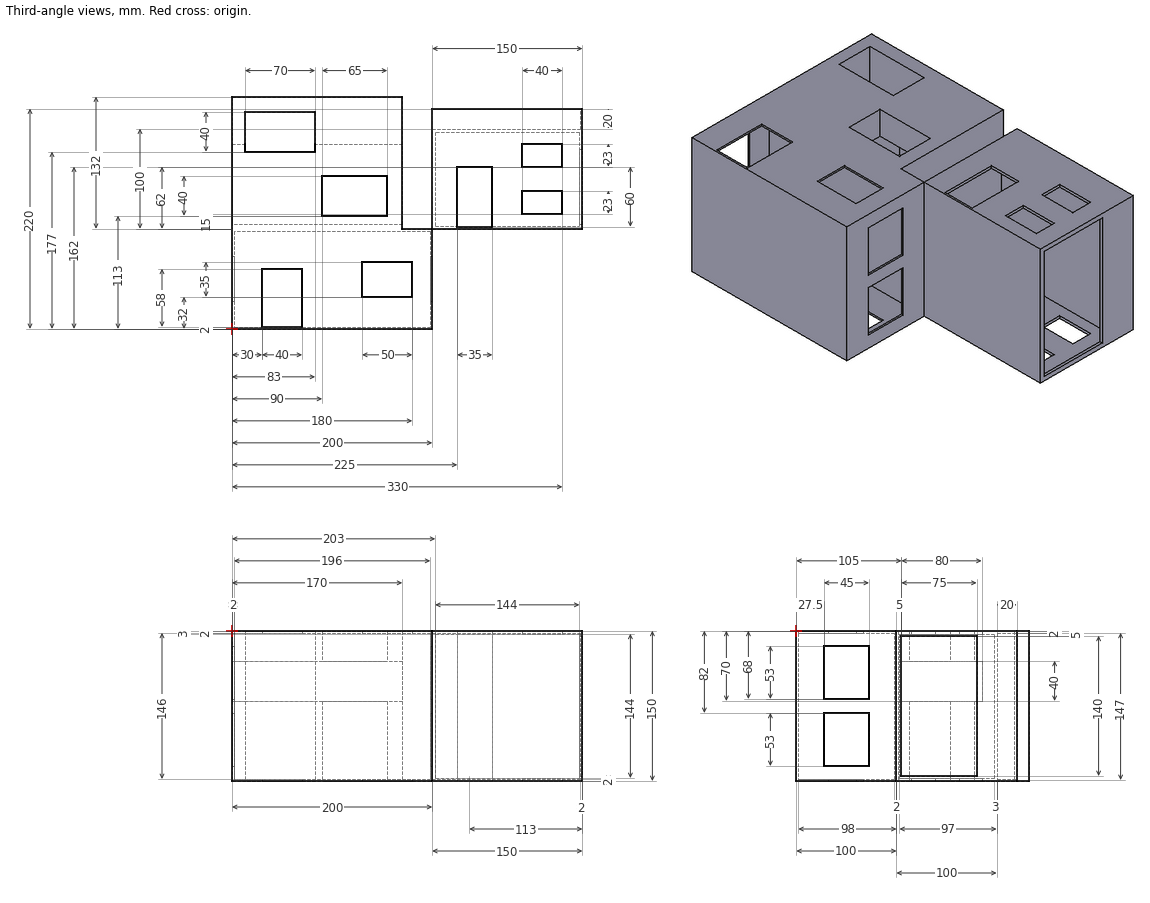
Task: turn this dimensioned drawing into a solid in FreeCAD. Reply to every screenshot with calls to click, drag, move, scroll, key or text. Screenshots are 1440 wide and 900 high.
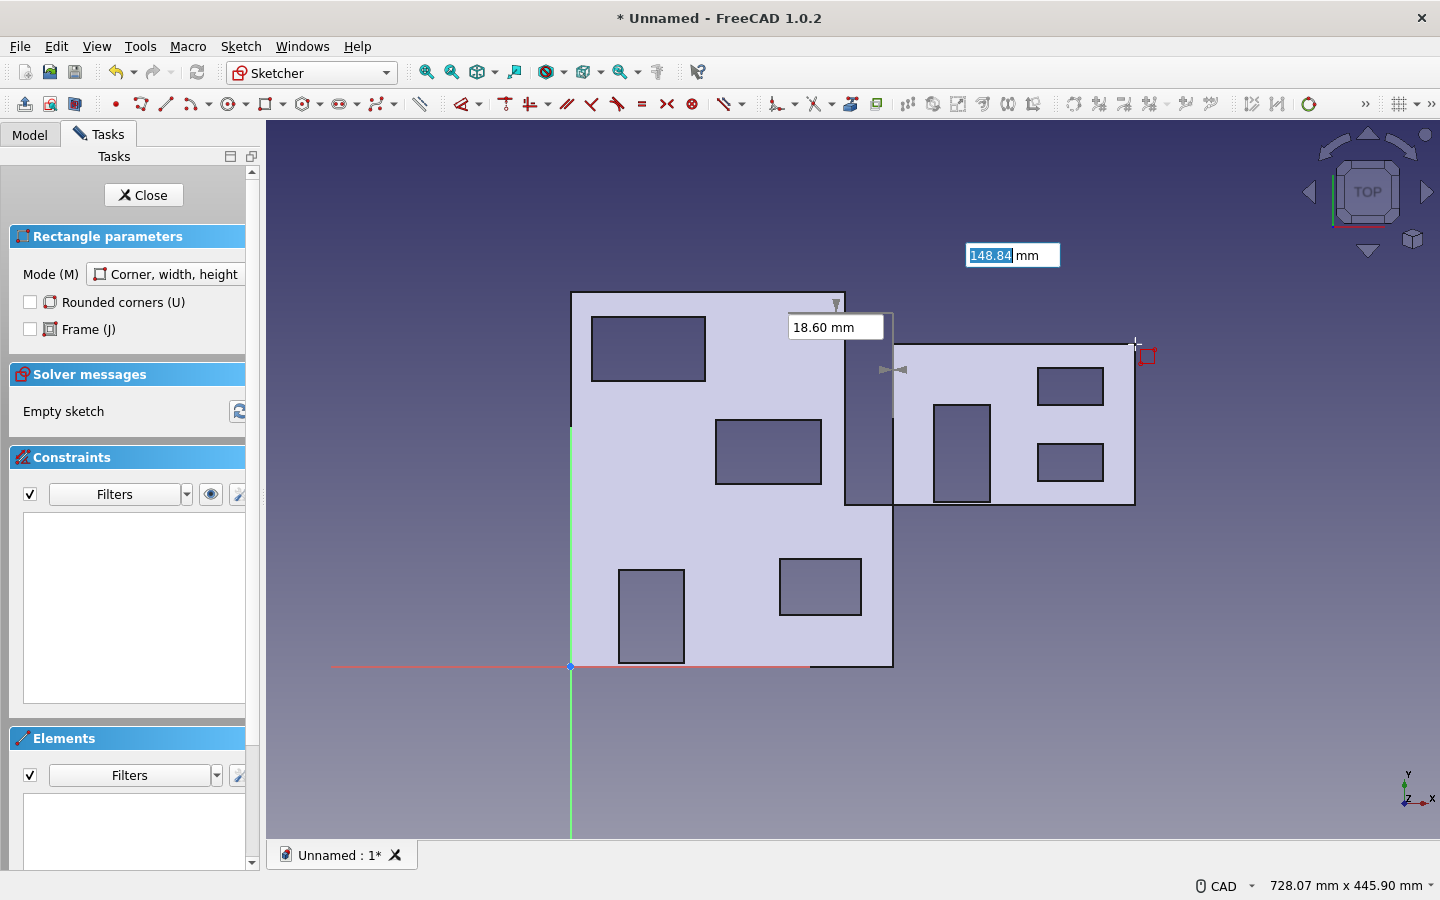
text(150)
key(Tab)
text(20)
key(Return)
key(Escape)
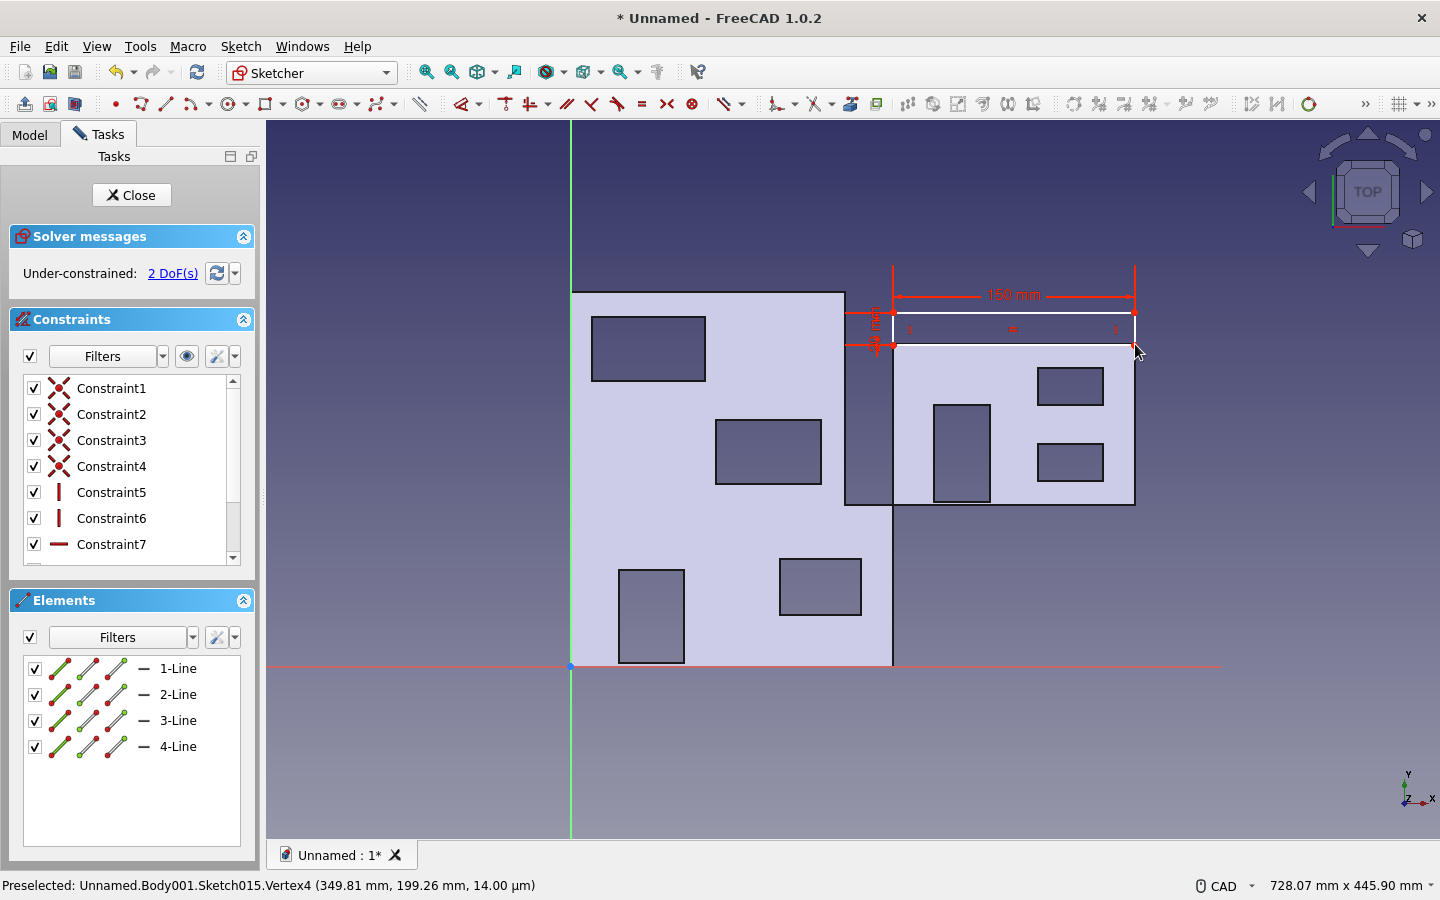
click(460, 104)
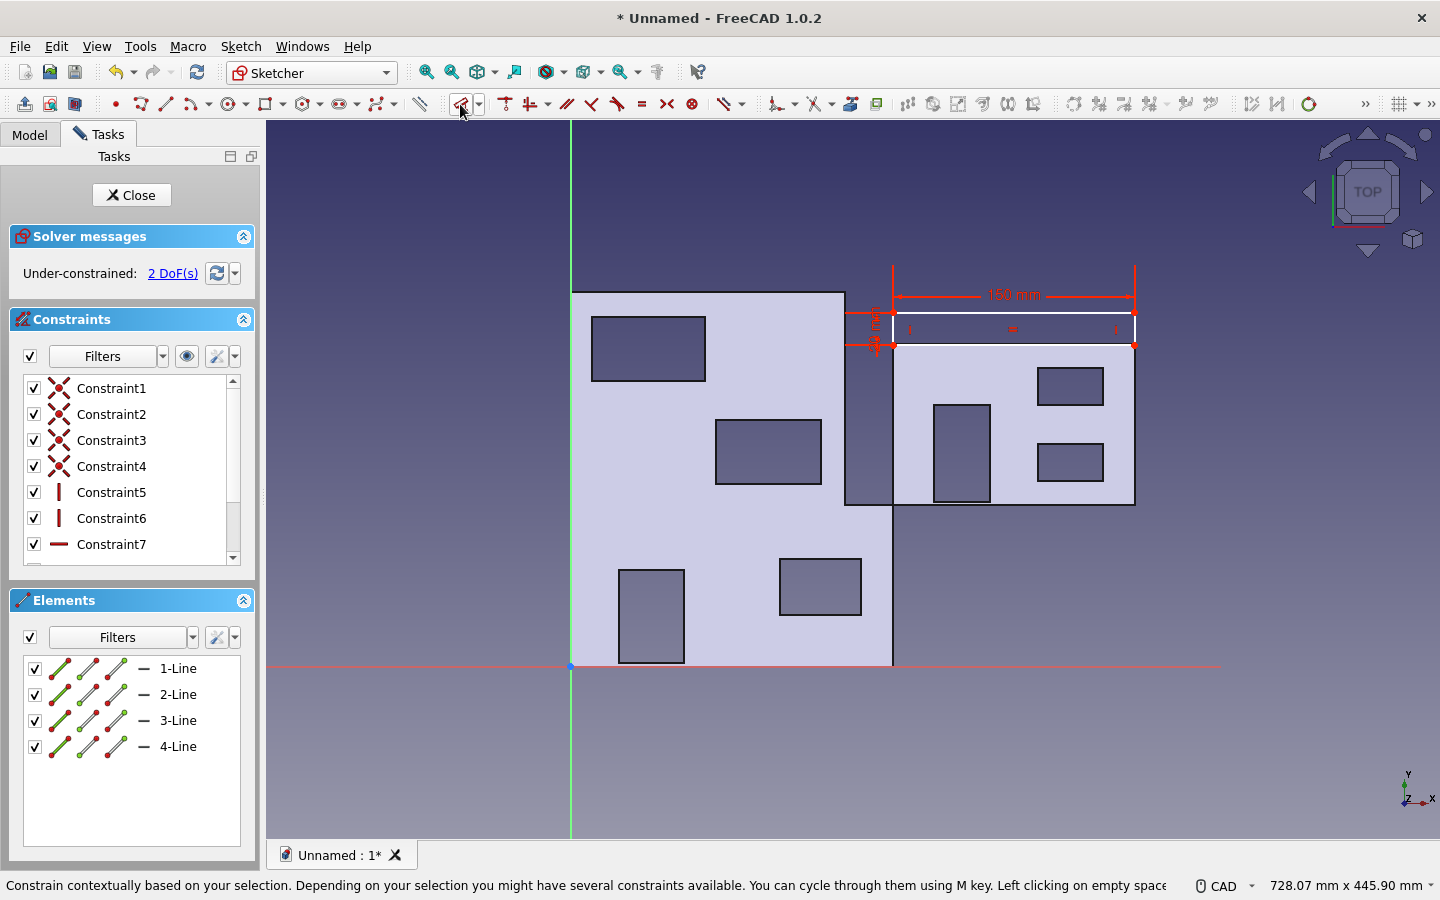
click(893, 313)
click(732, 701)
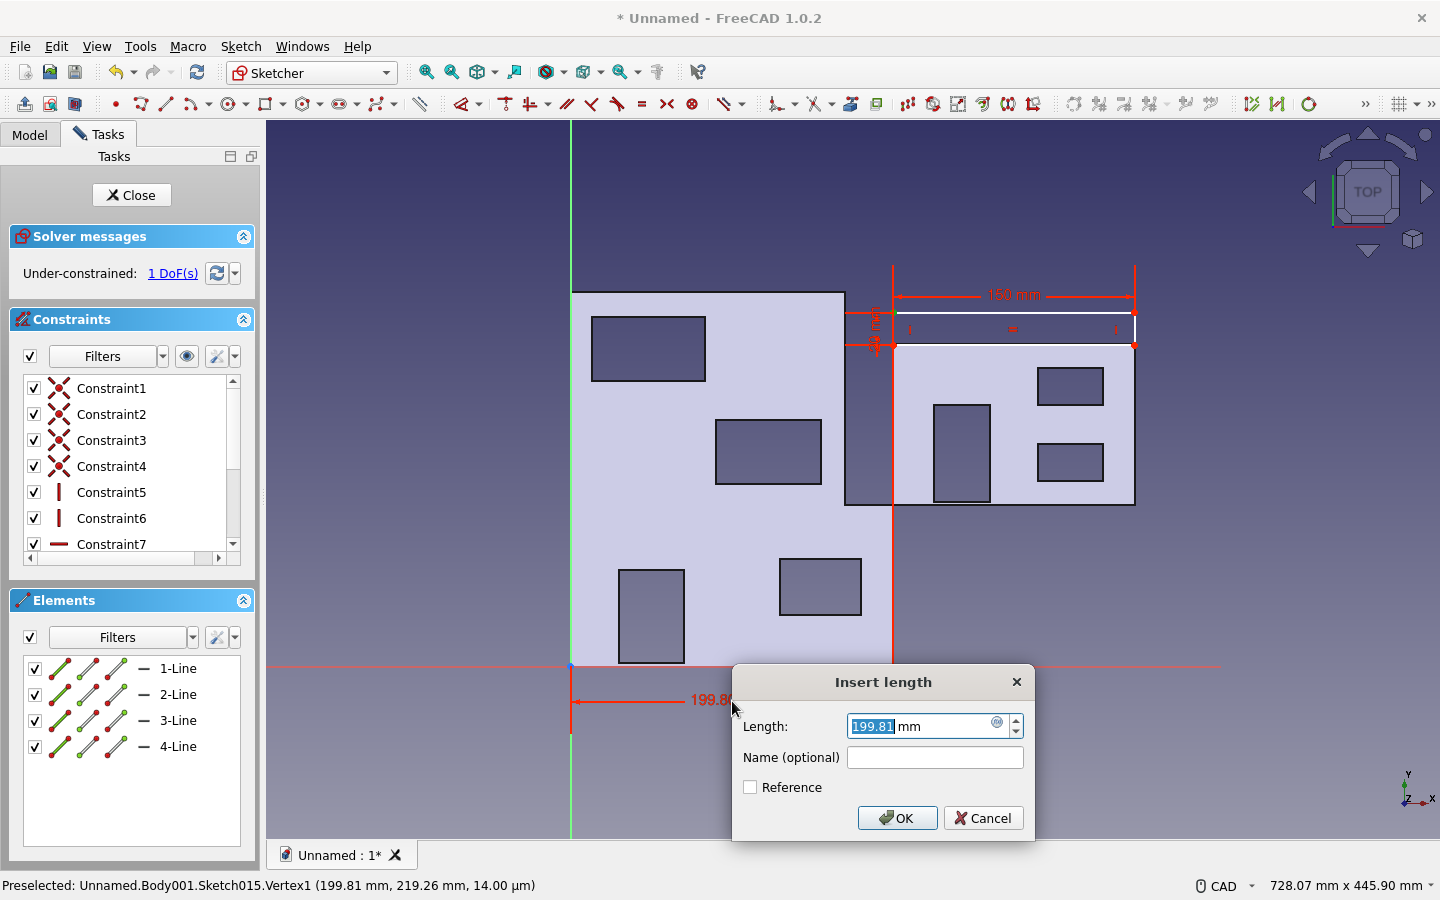
text(200)
key(Return)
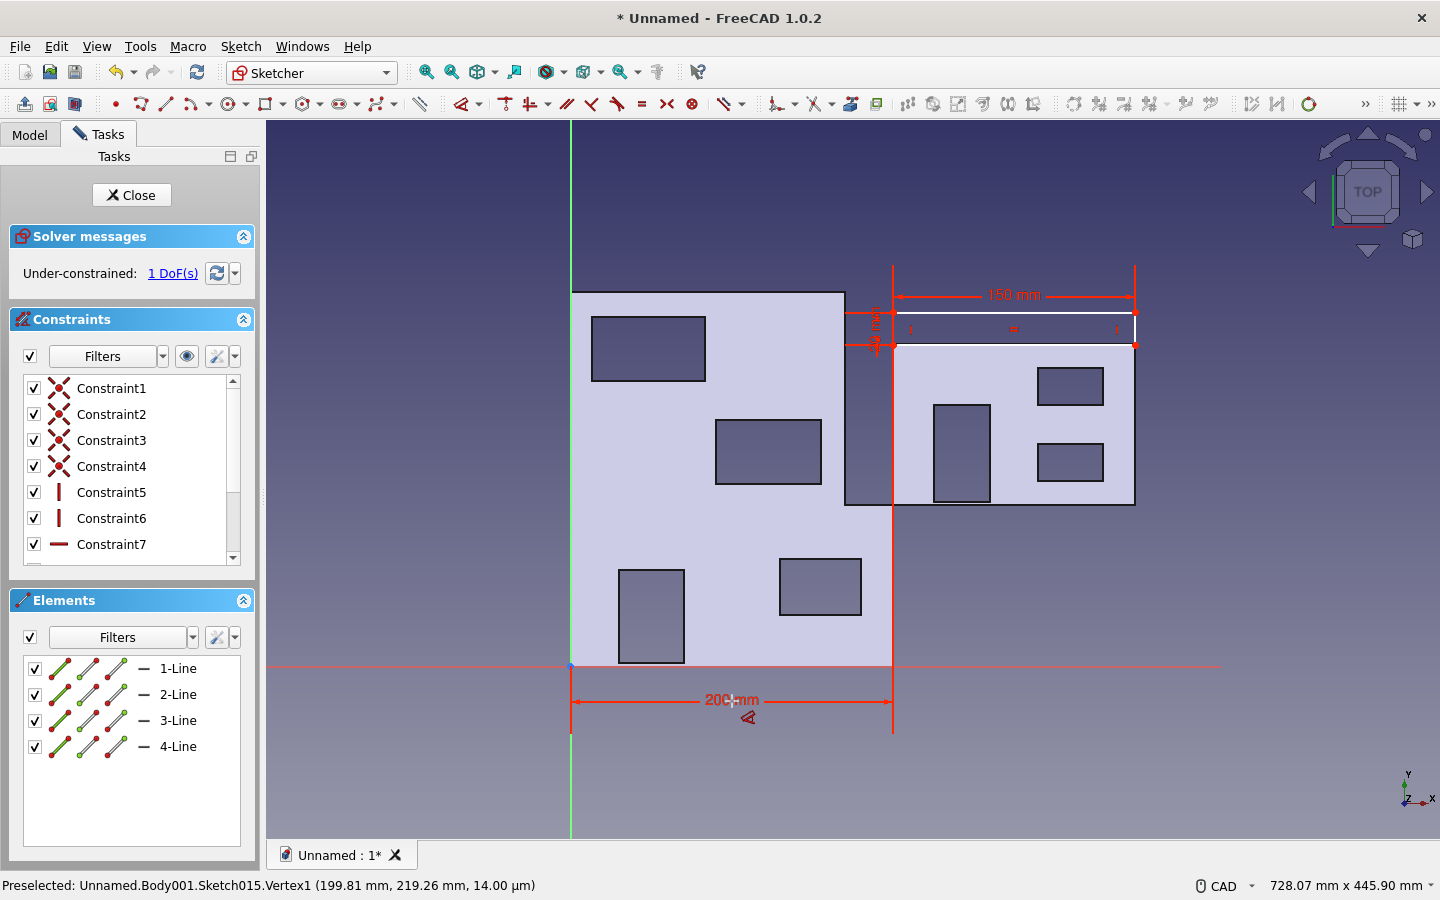
click(893, 313)
click(537, 490)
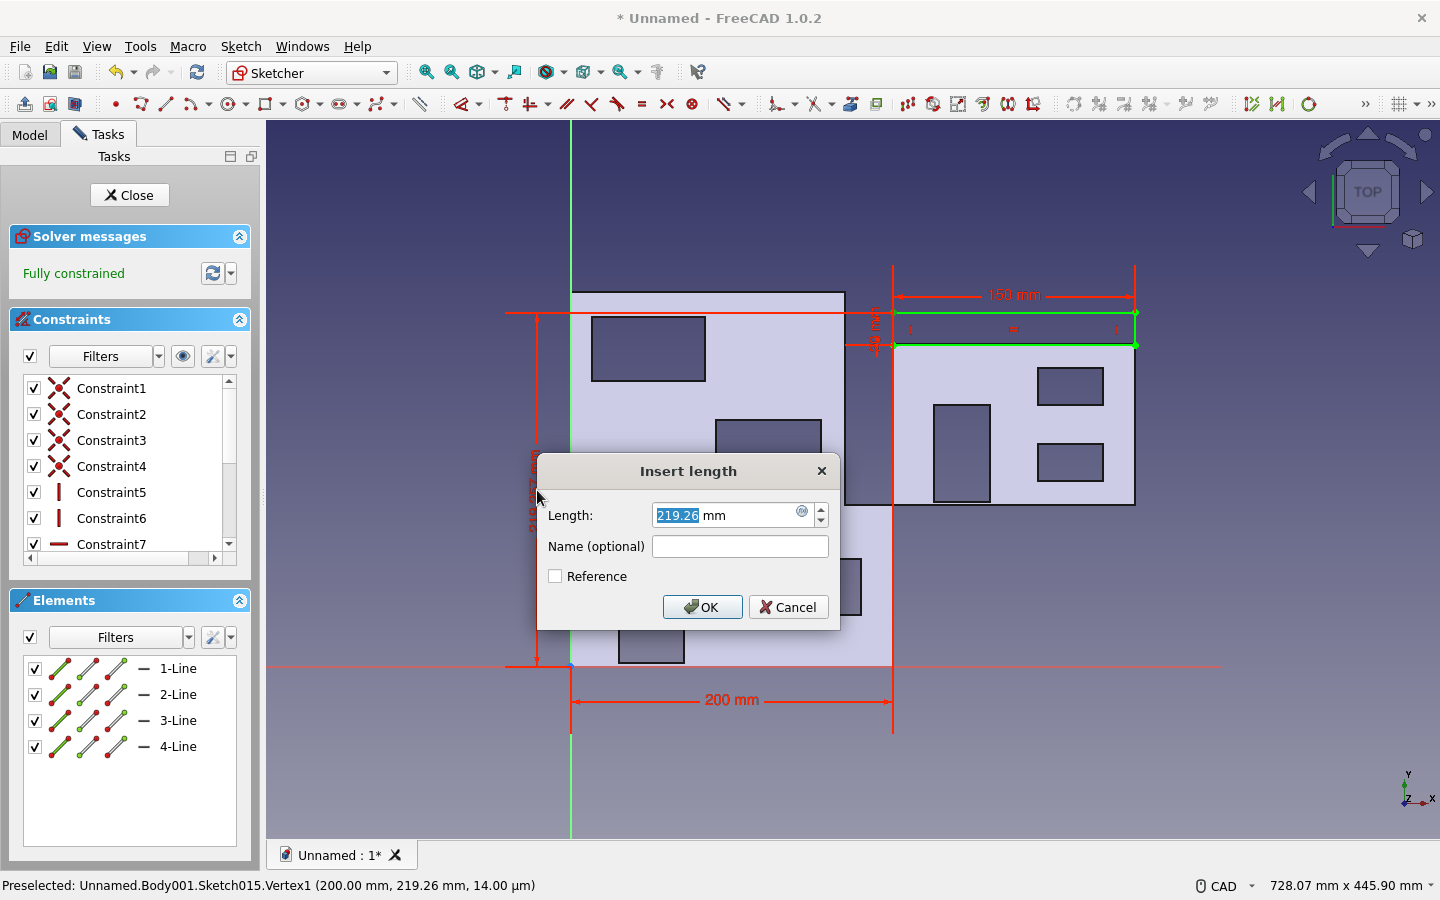
text(220)
key(Return)
key(Escape)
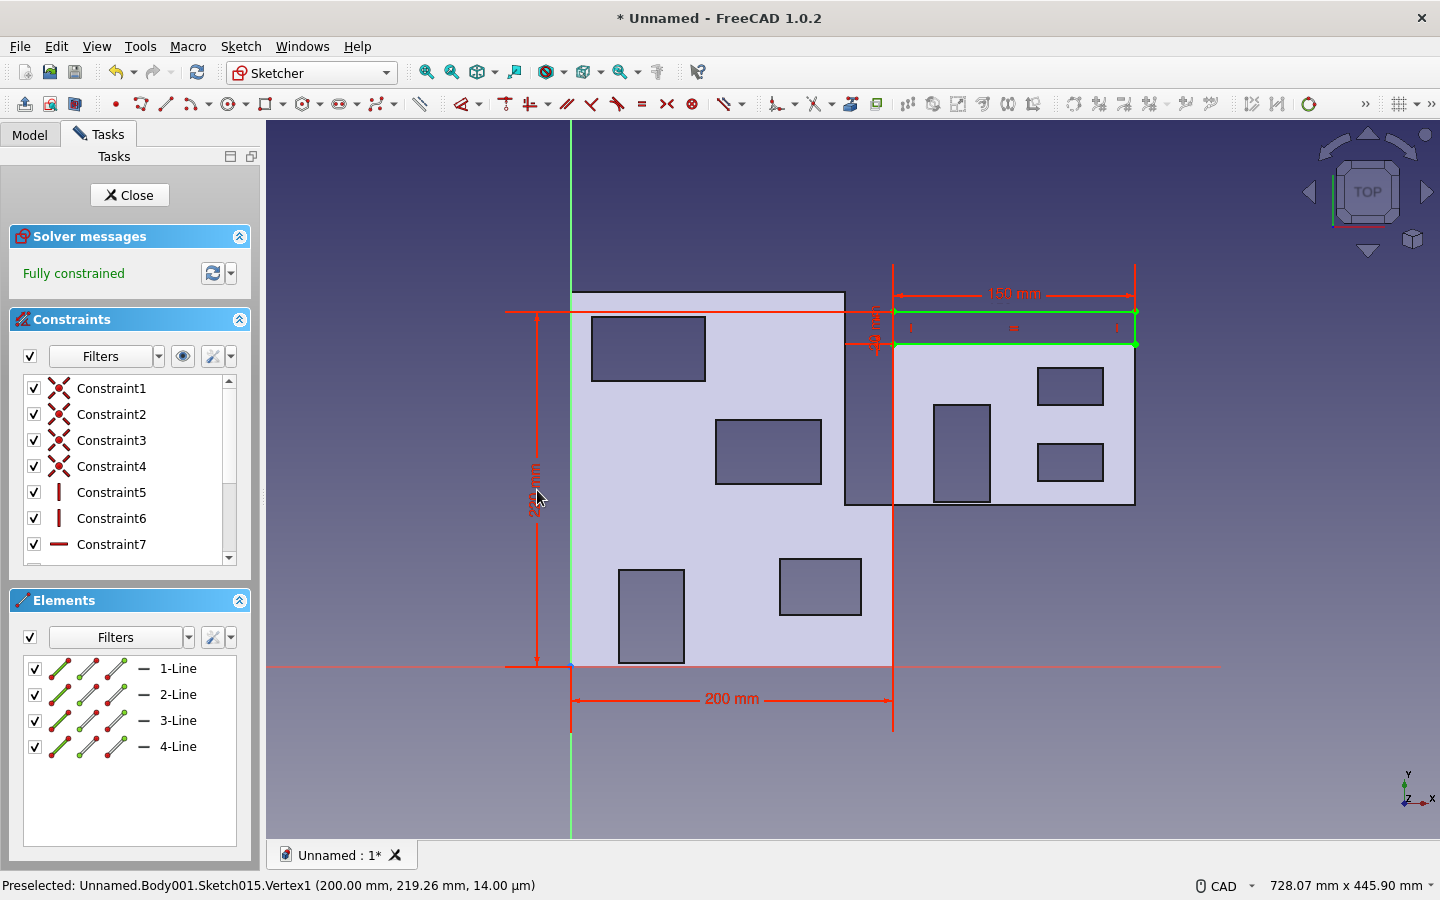
click(130, 195)